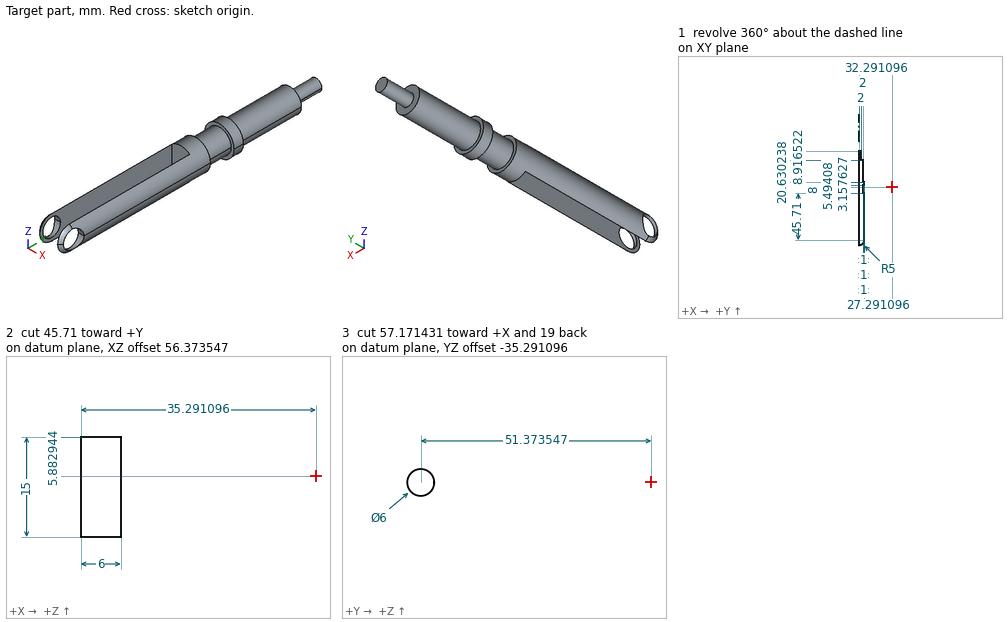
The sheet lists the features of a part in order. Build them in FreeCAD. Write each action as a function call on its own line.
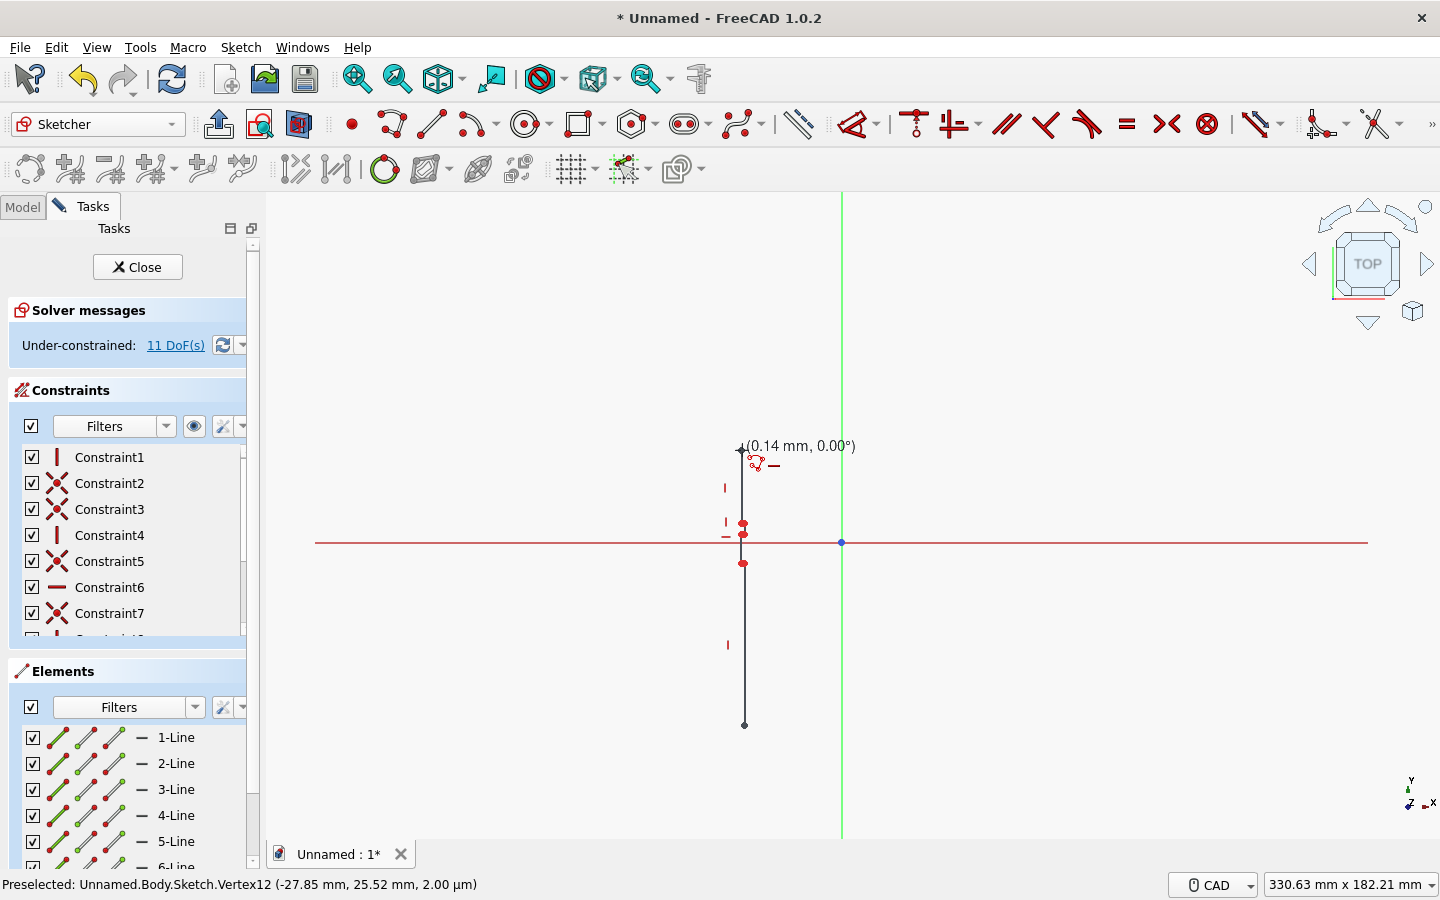
scroll(734, 450, up, 5)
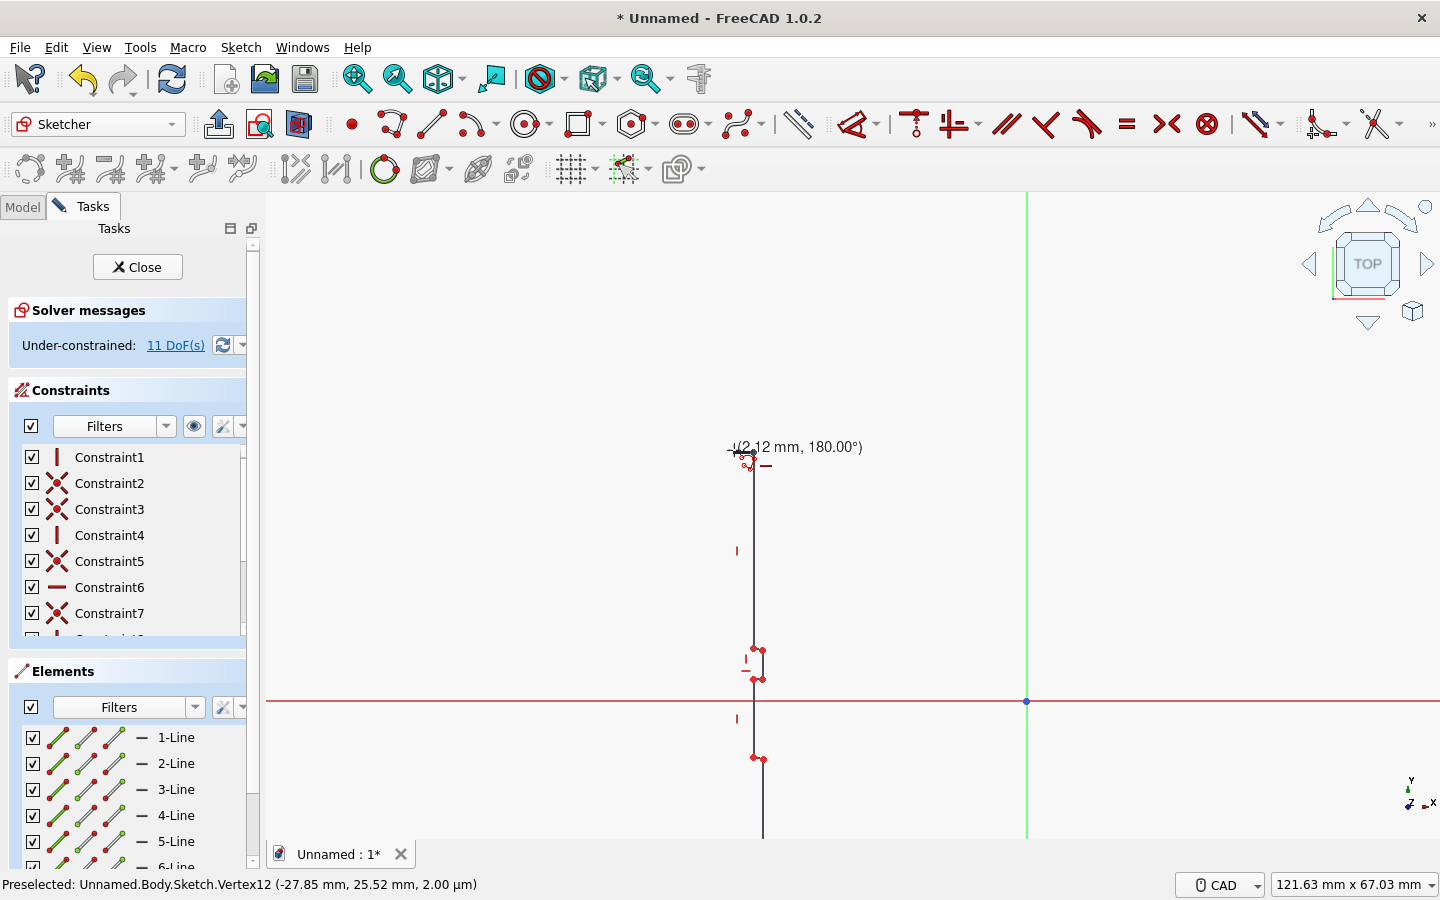
click(734, 449)
click(734, 363)
click(715, 363)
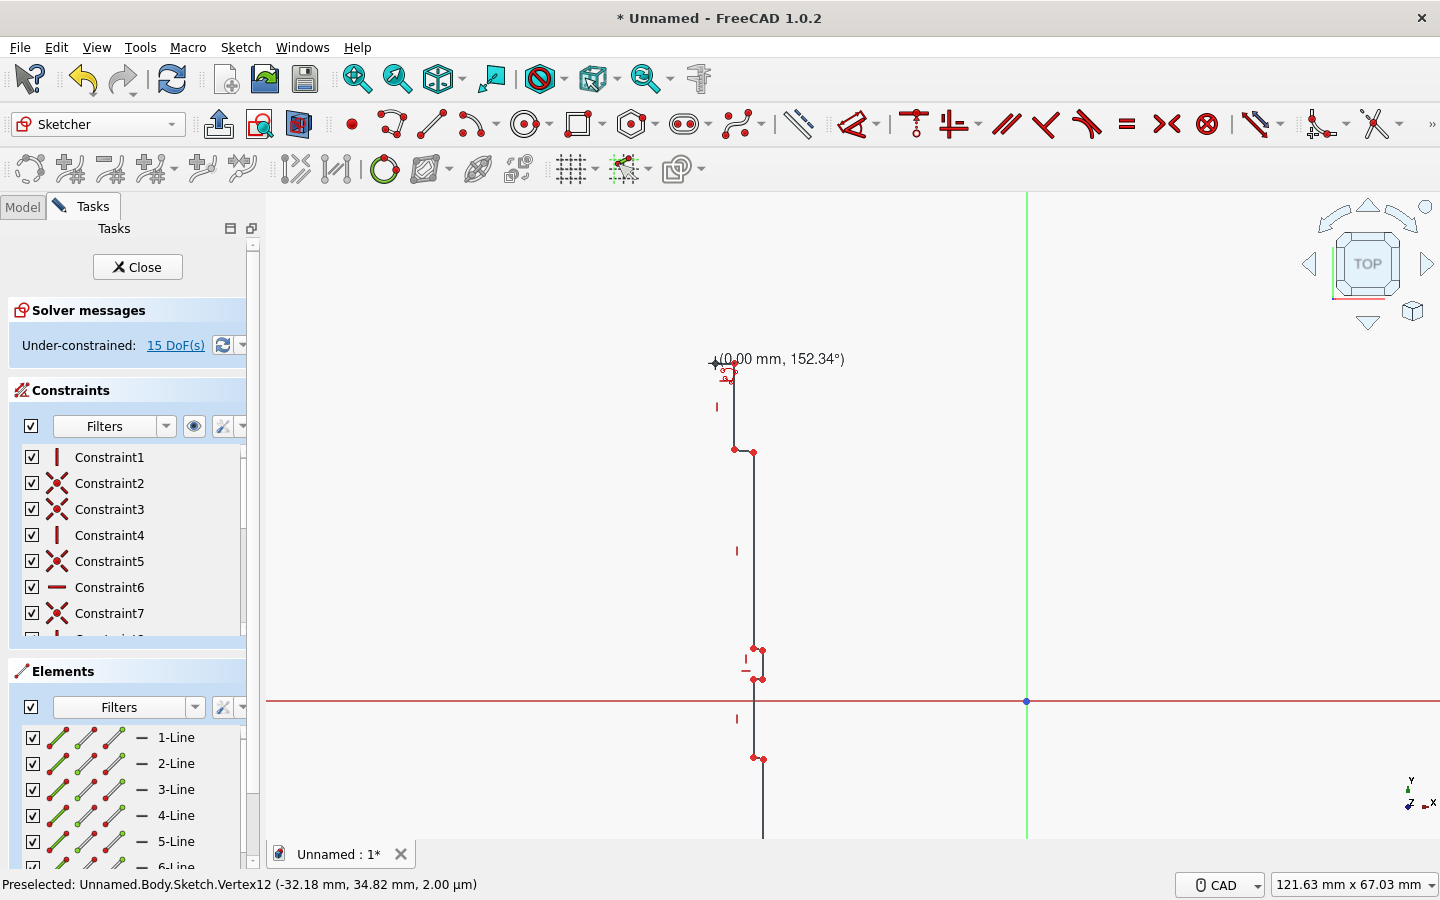
scroll(734, 450, down, 5)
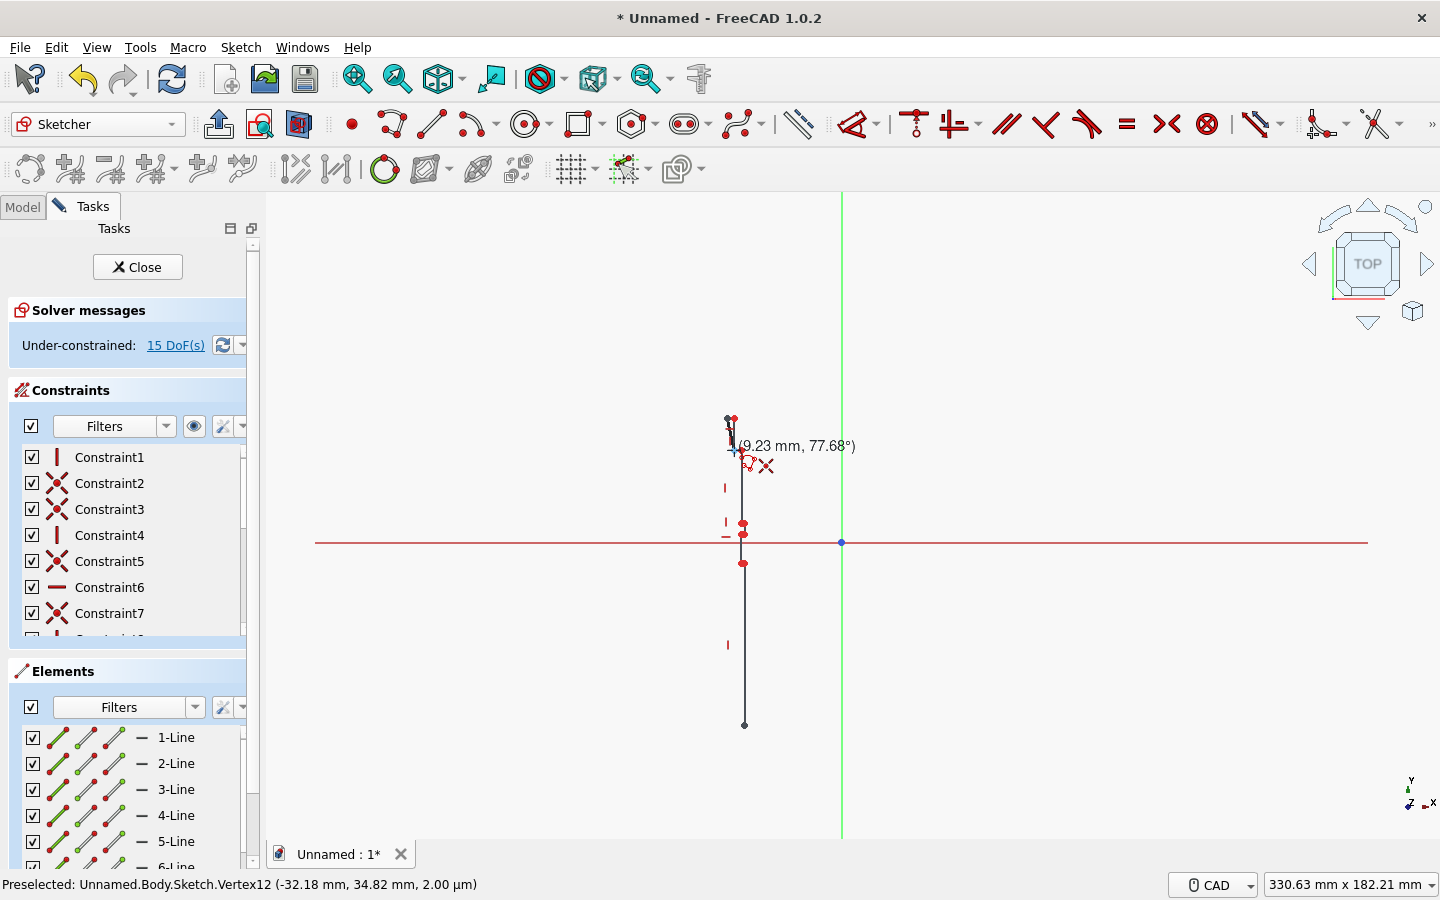
click(727, 743)
right_click(727, 743)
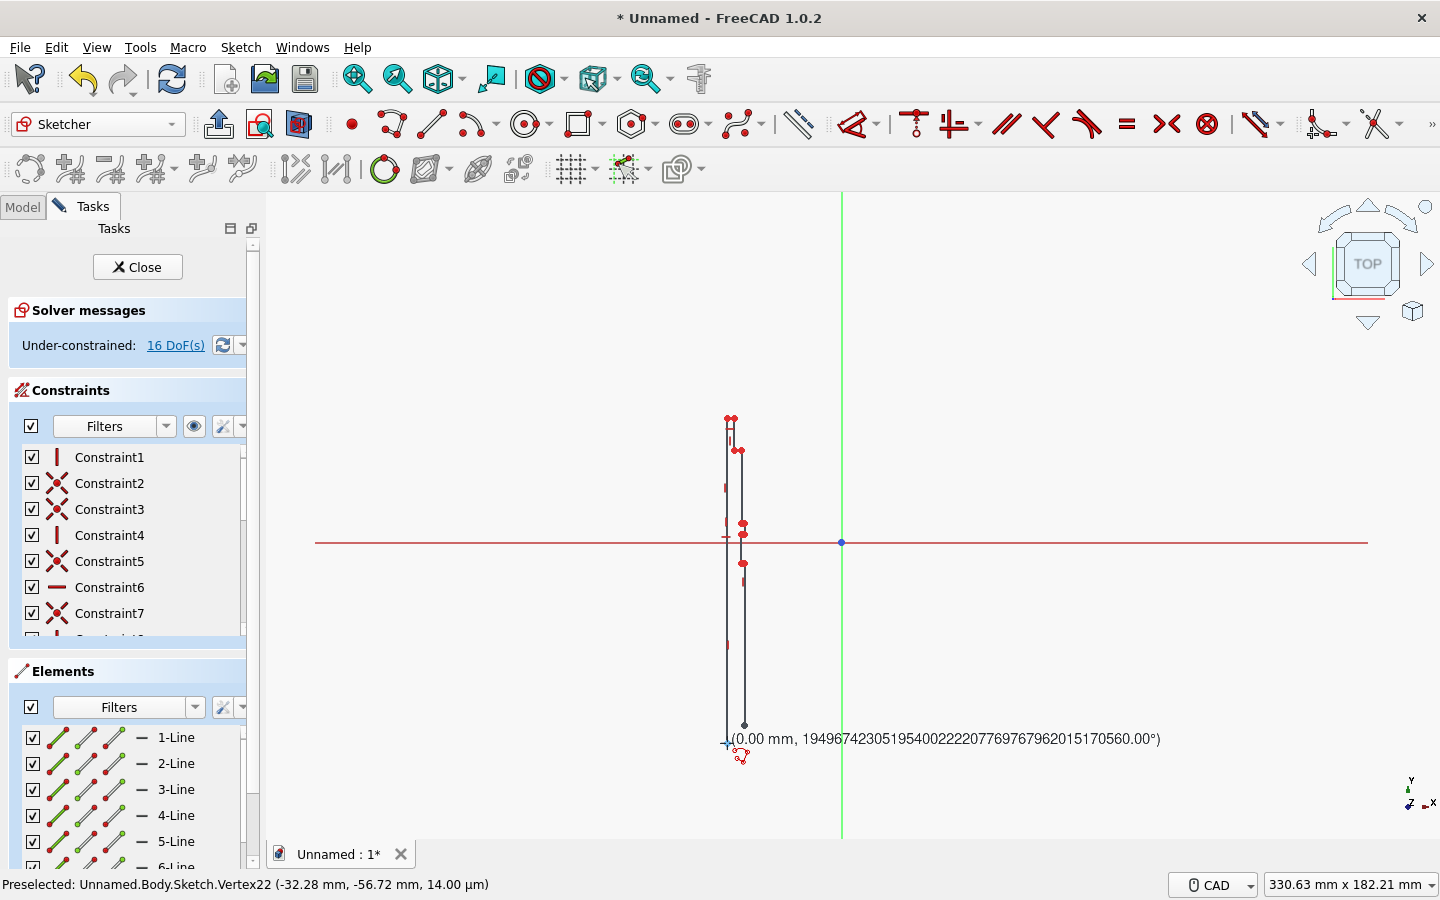
click(498, 124)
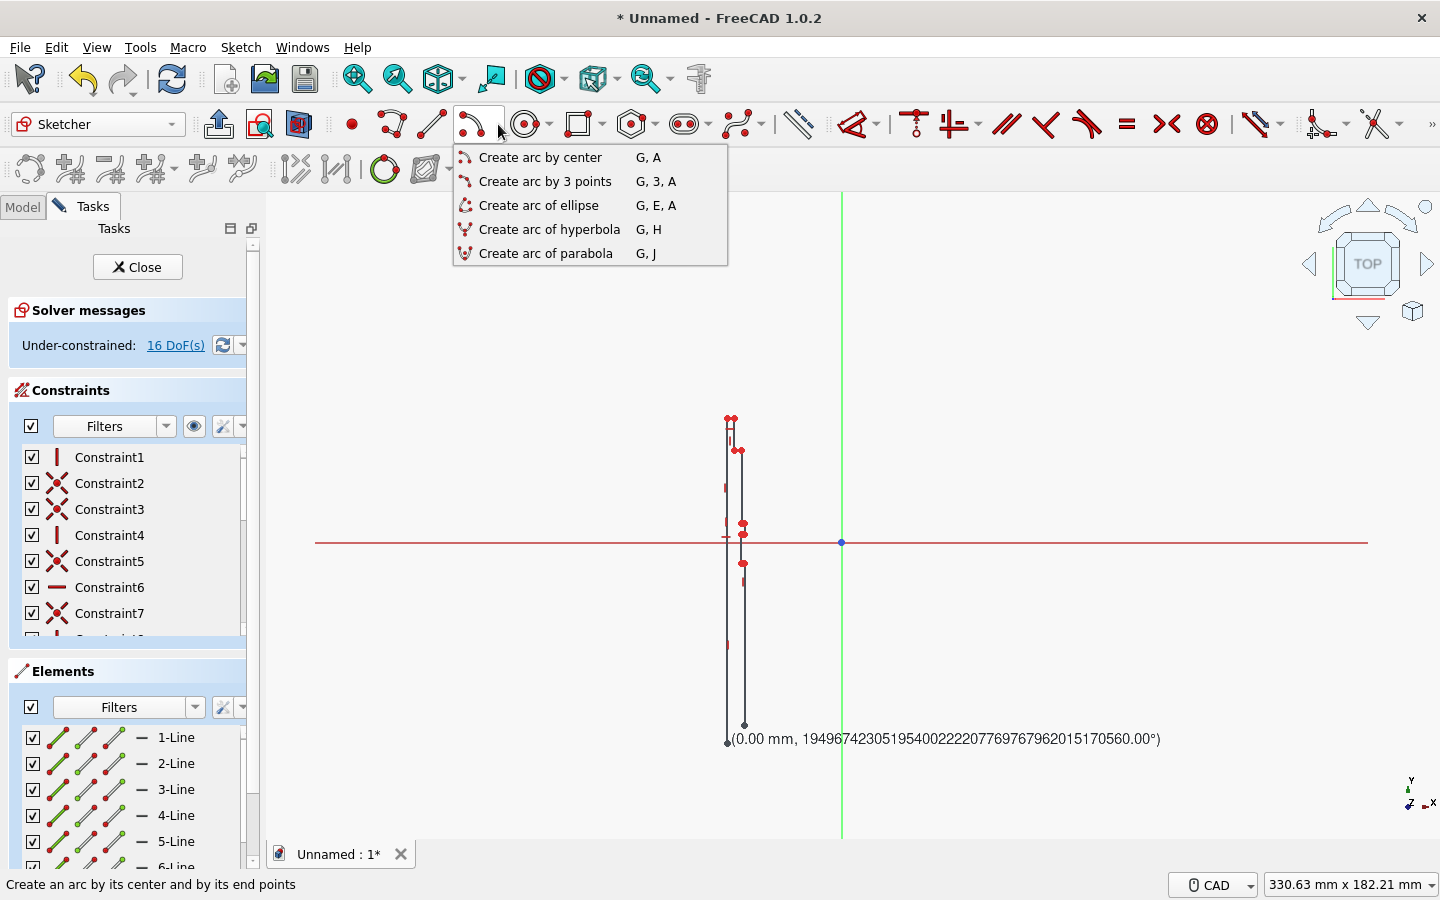
click(590, 181)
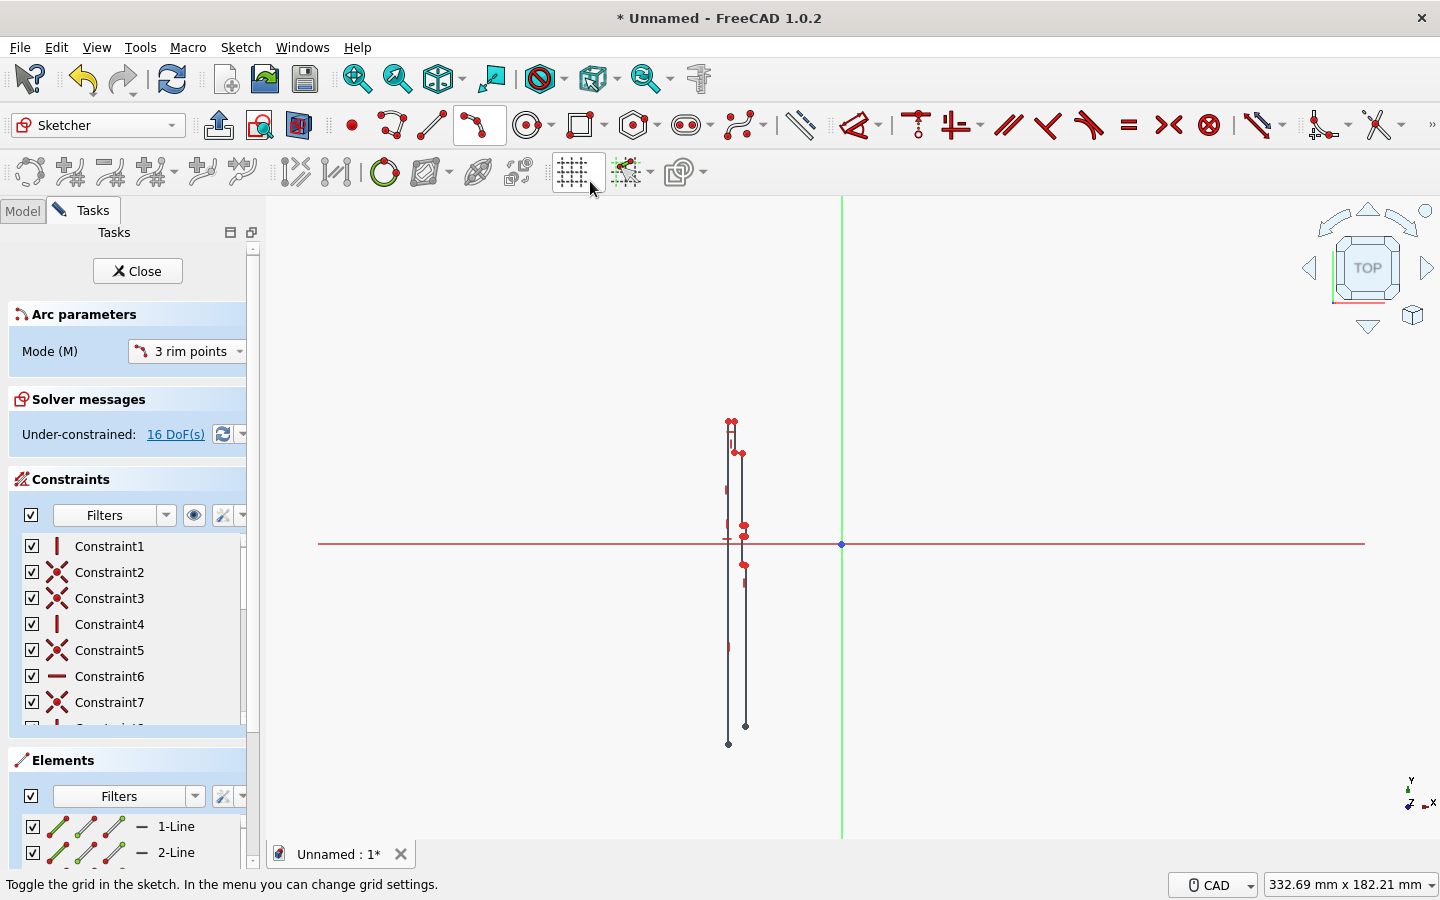
click(728, 745)
click(746, 727)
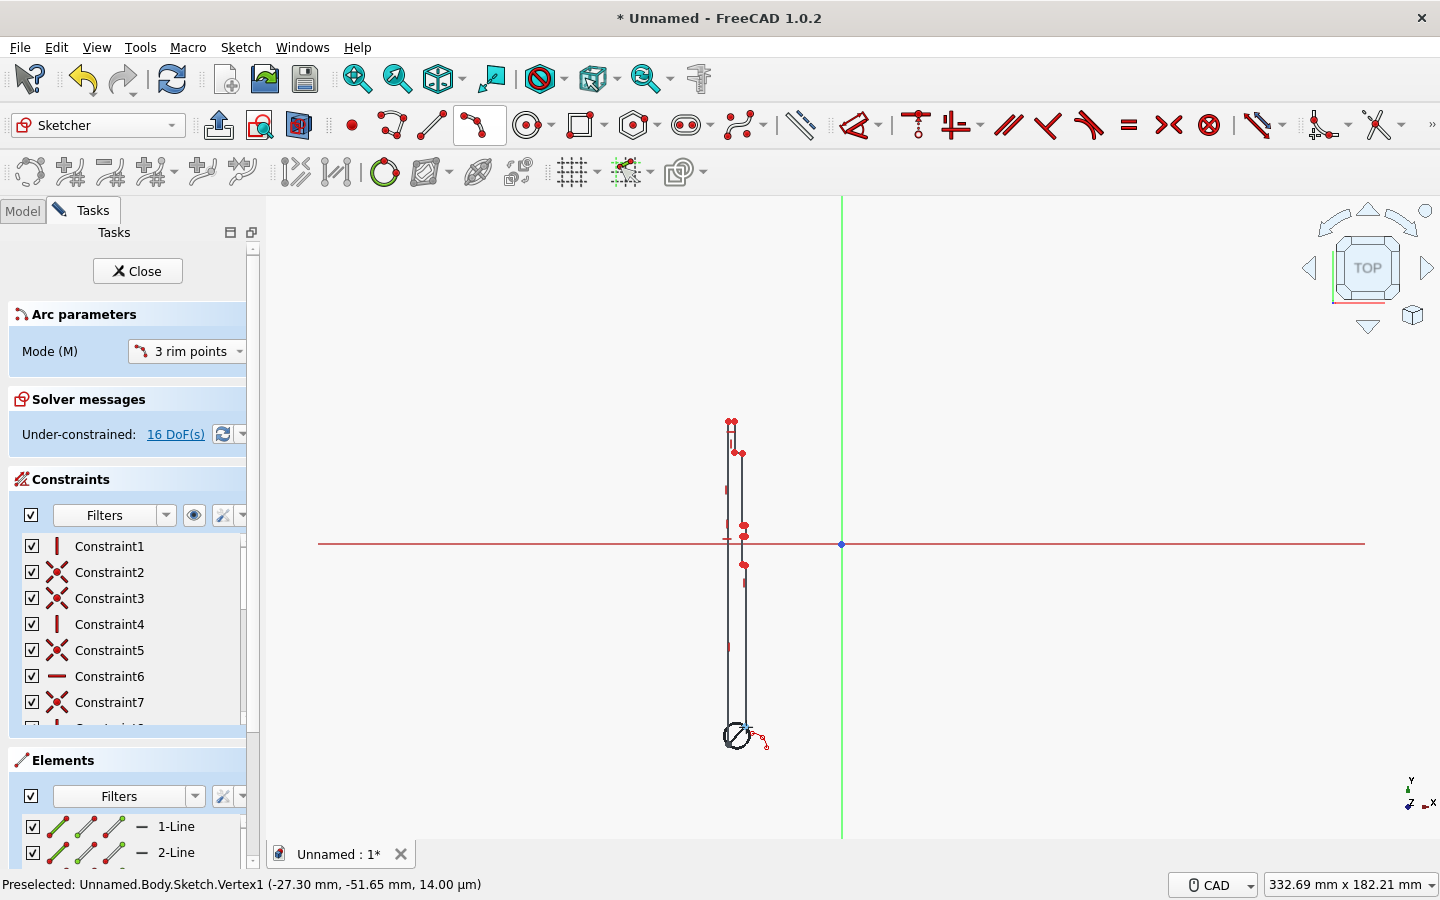
scroll(740, 738, up, 6)